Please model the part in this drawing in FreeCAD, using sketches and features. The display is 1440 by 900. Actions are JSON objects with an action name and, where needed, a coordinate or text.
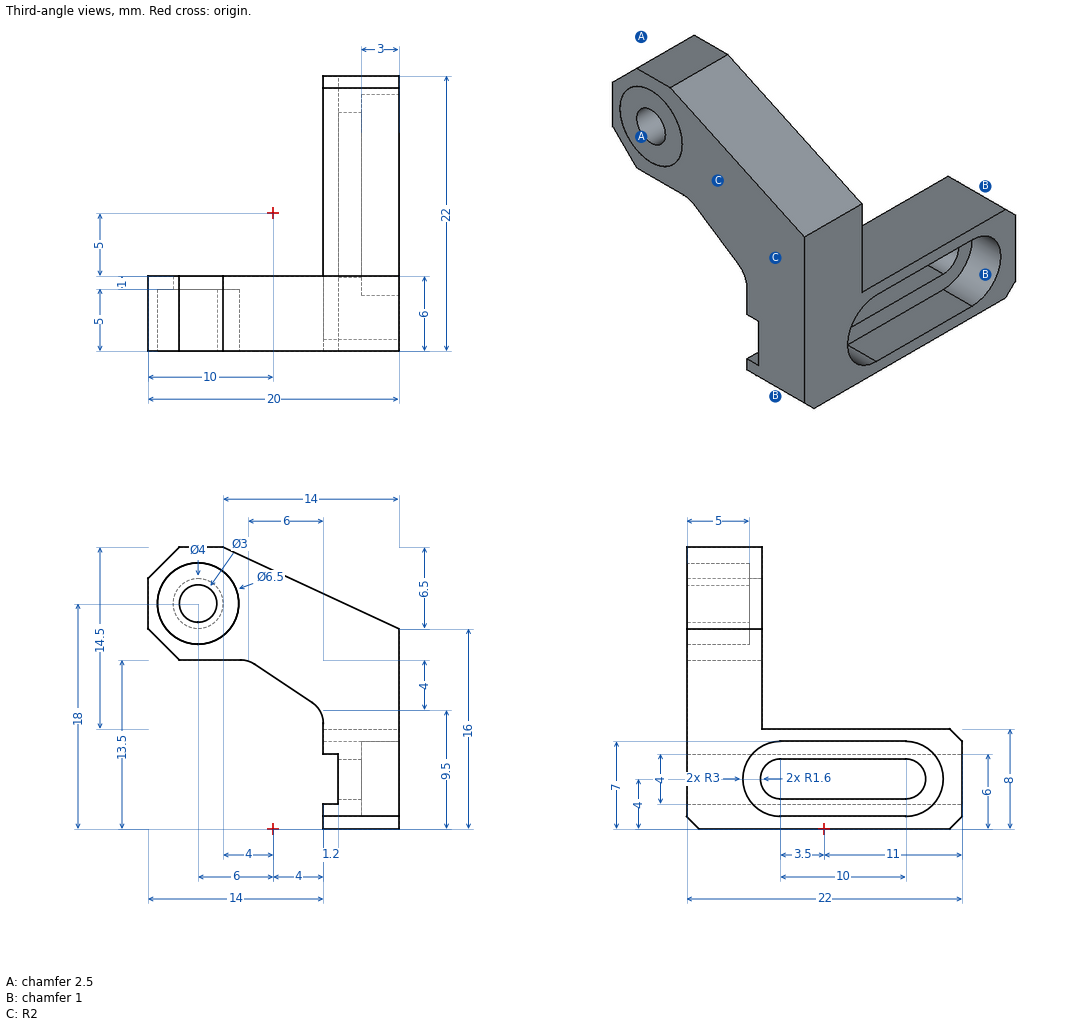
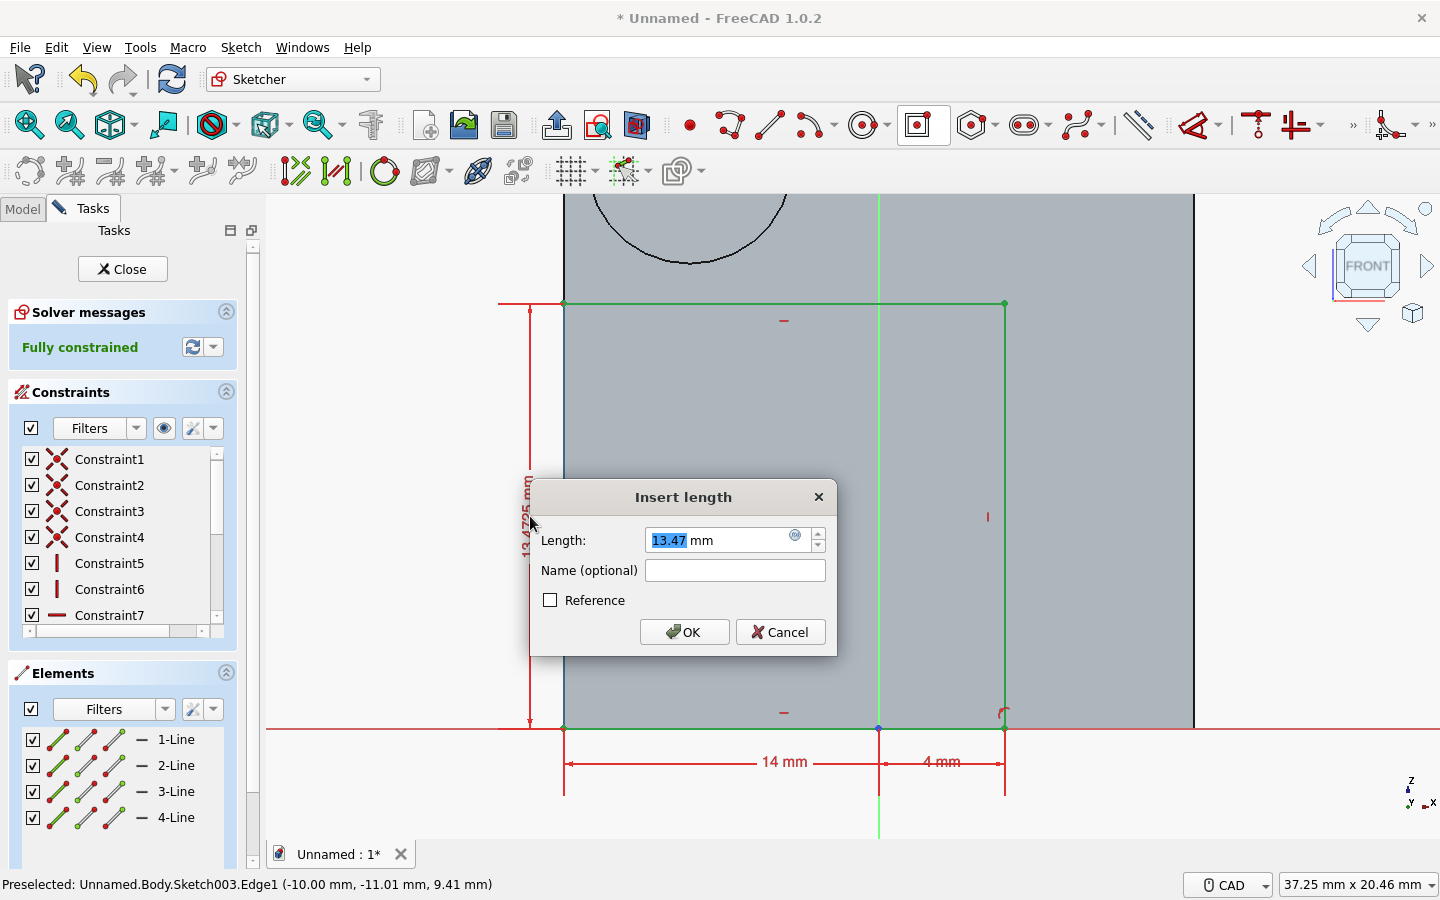
{"action": "type", "text": "13.5"}
{"action": "key", "text": "Return"}
{"action": "key", "text": "Escape"}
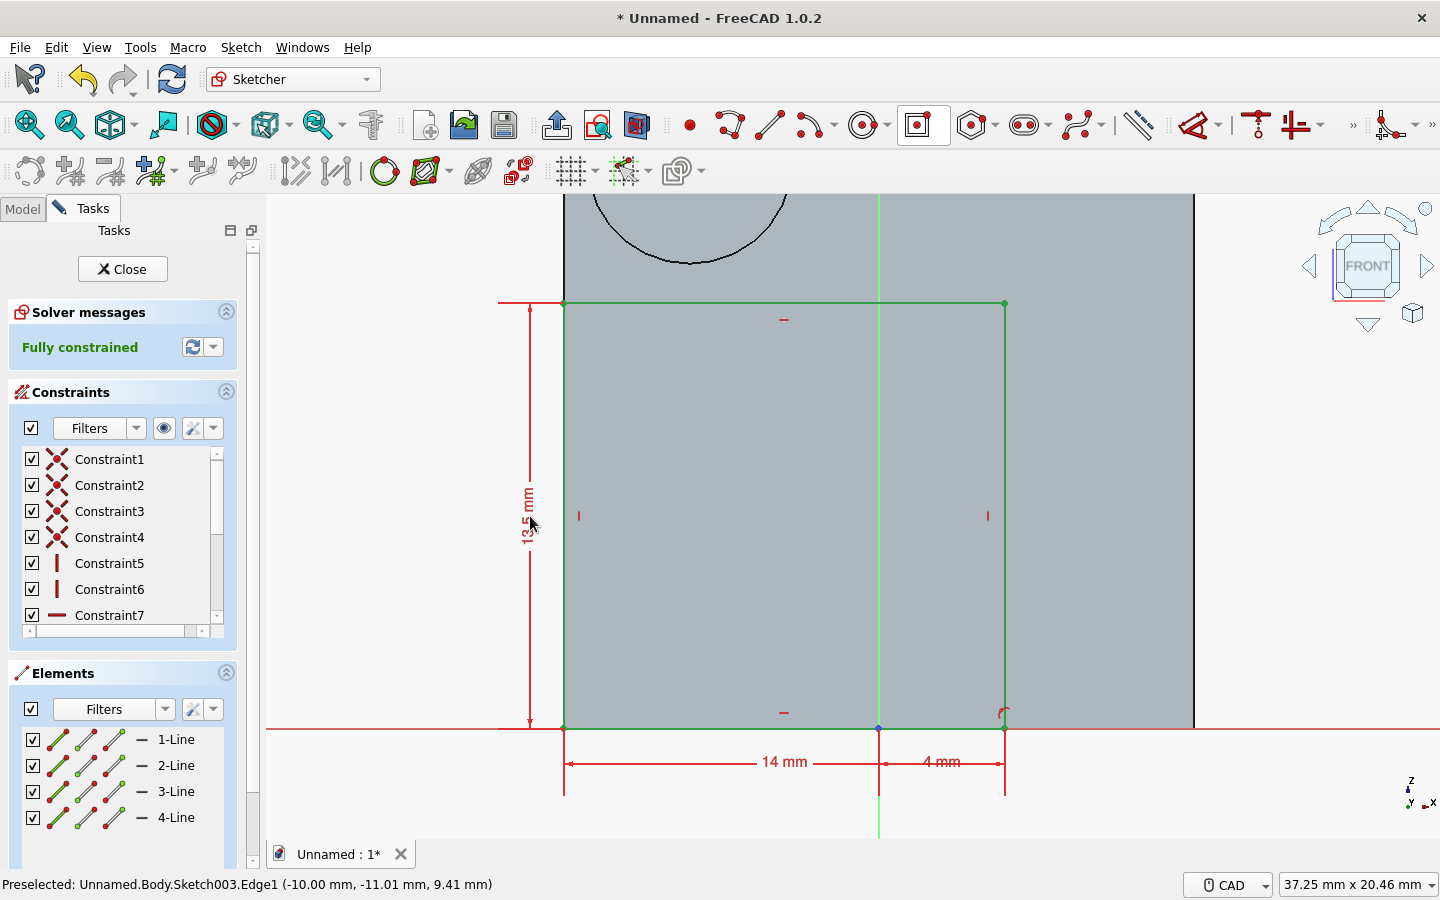
{"action": "left_click", "coordinate": [123, 269]}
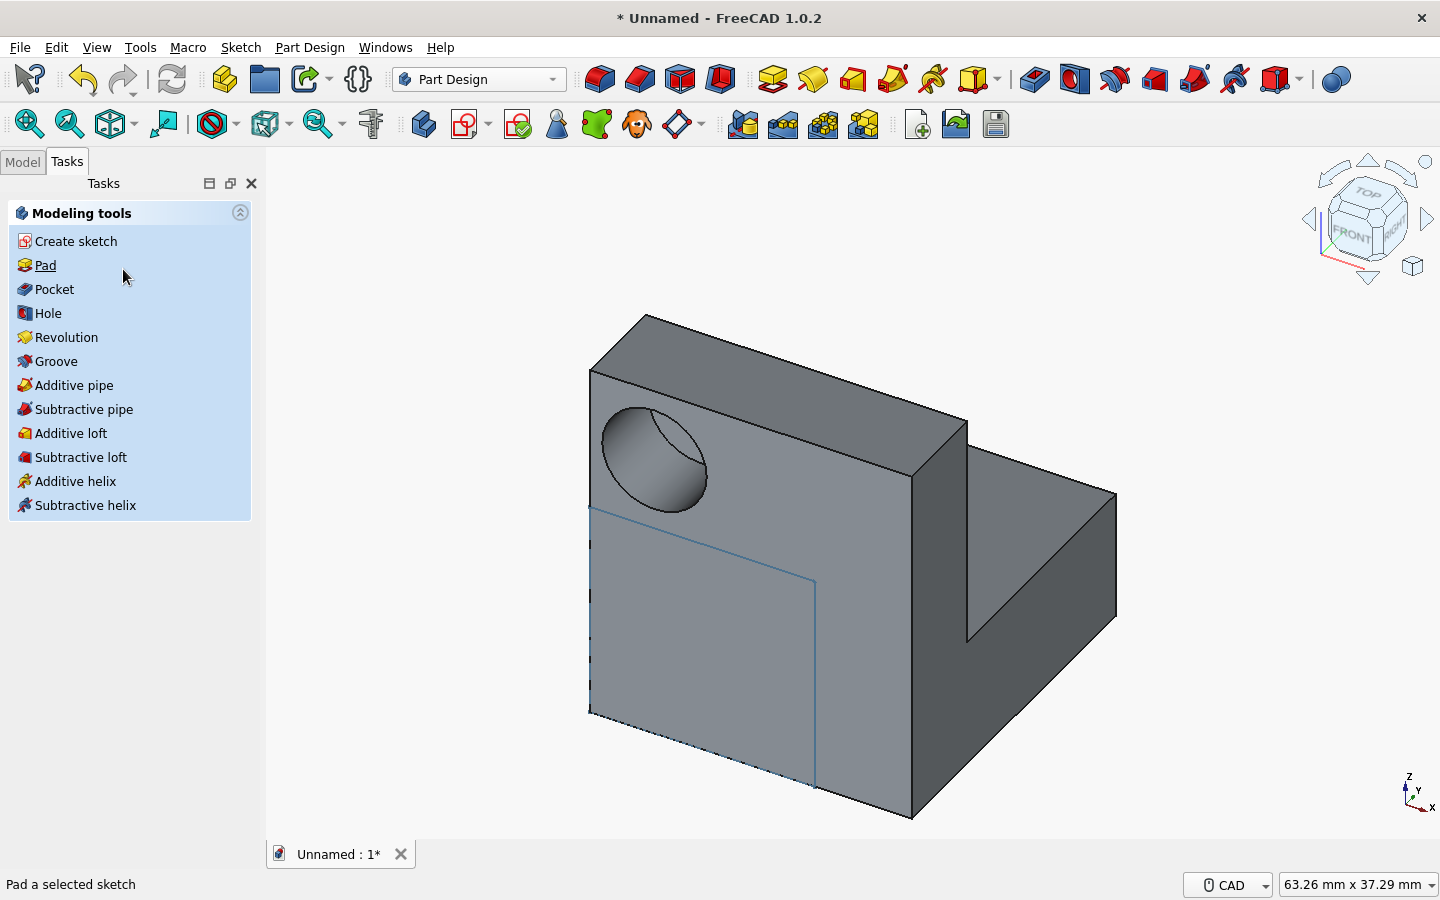
{"action": "left_click", "coordinate": [1036, 80]}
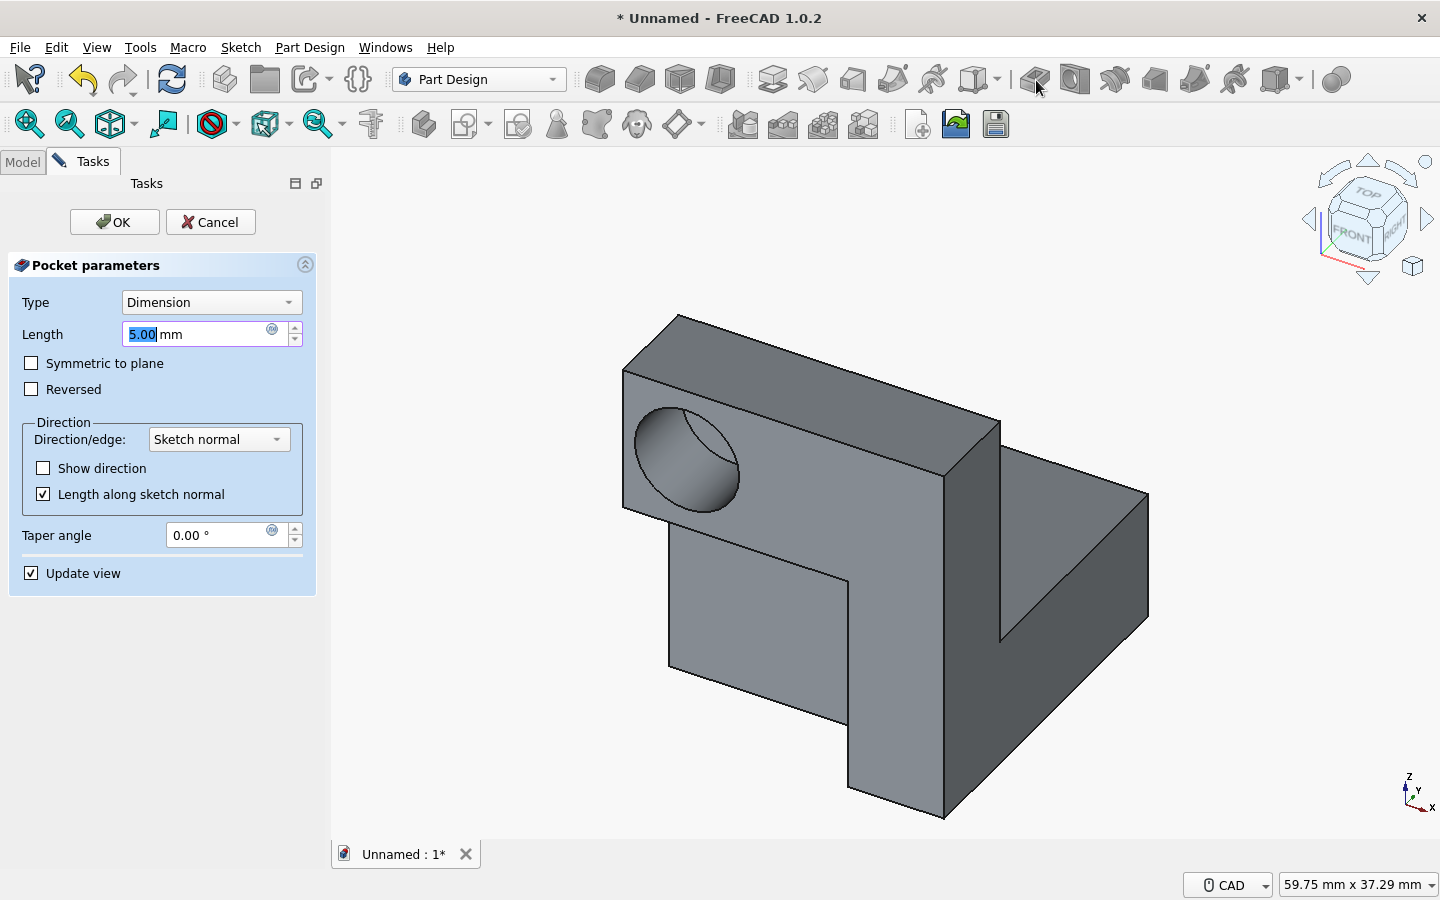
{"action": "left_click", "coordinate": [212, 302]}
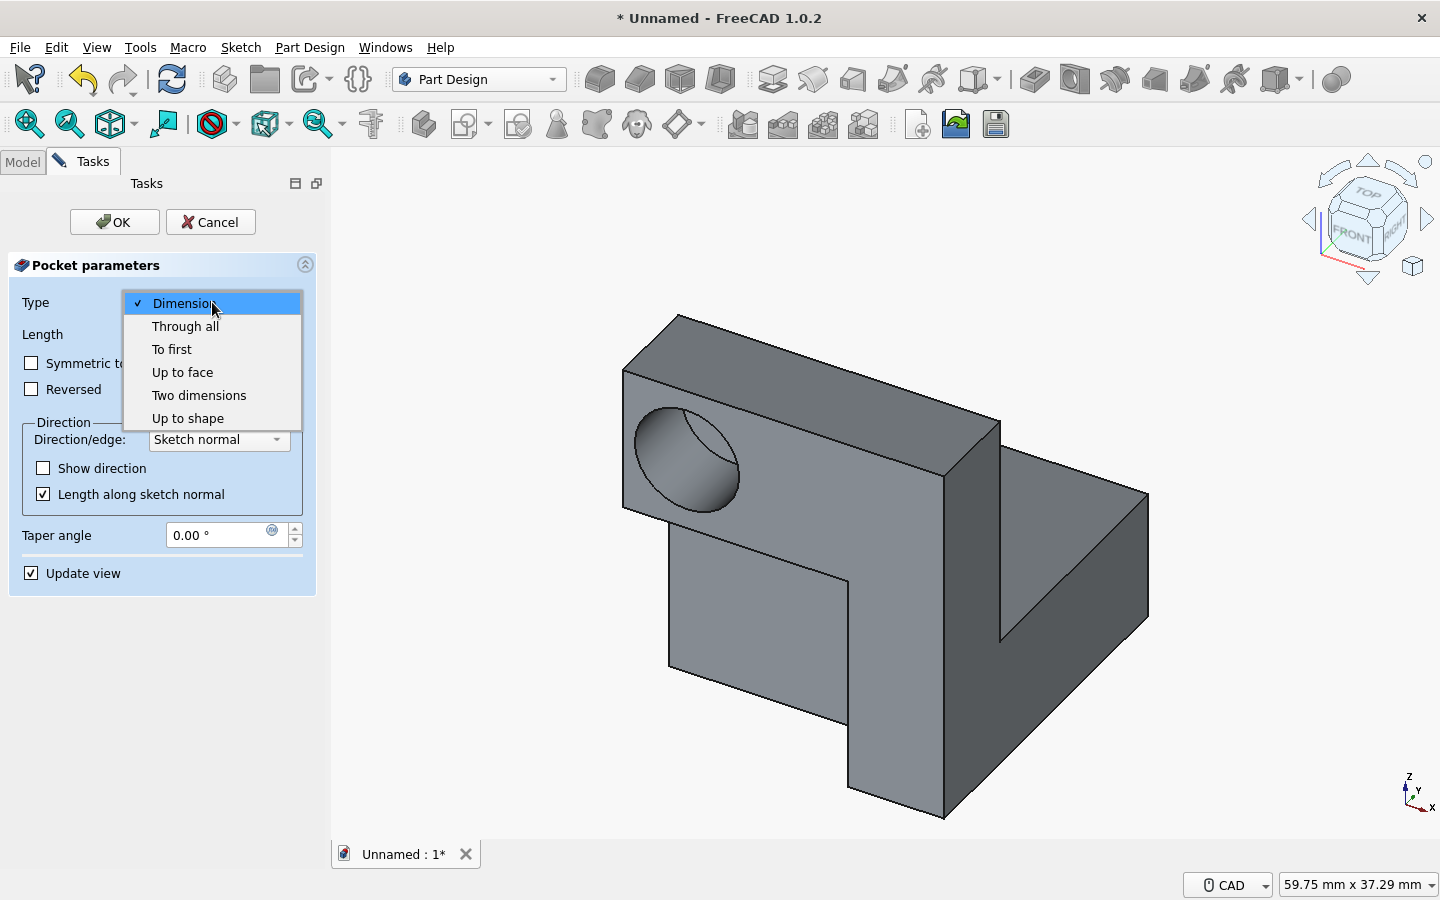
{"action": "left_click", "coordinate": [212, 326]}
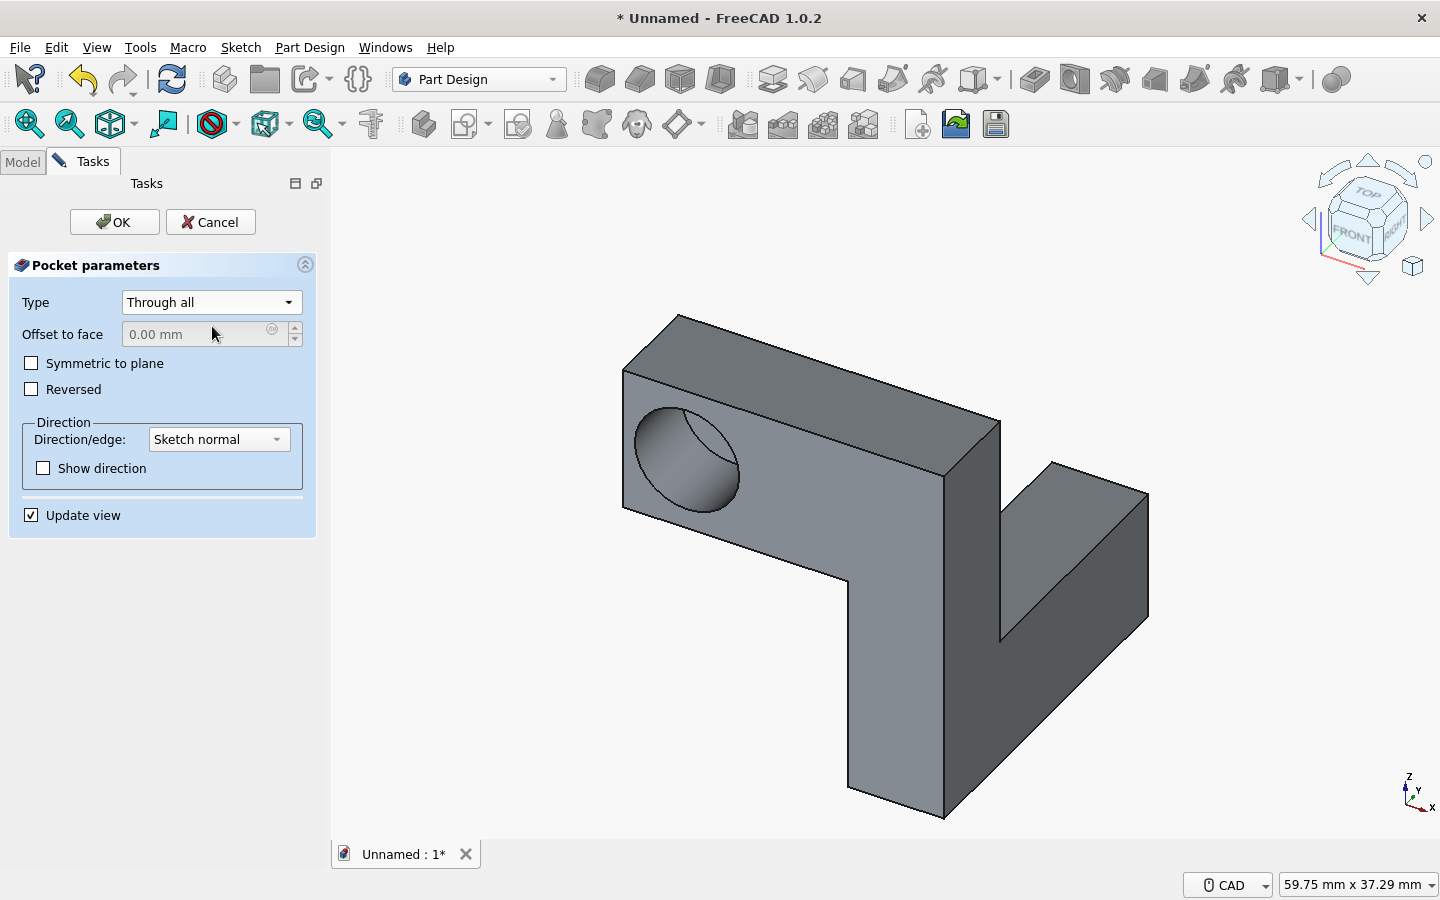
{"action": "left_click", "coordinate": [115, 222]}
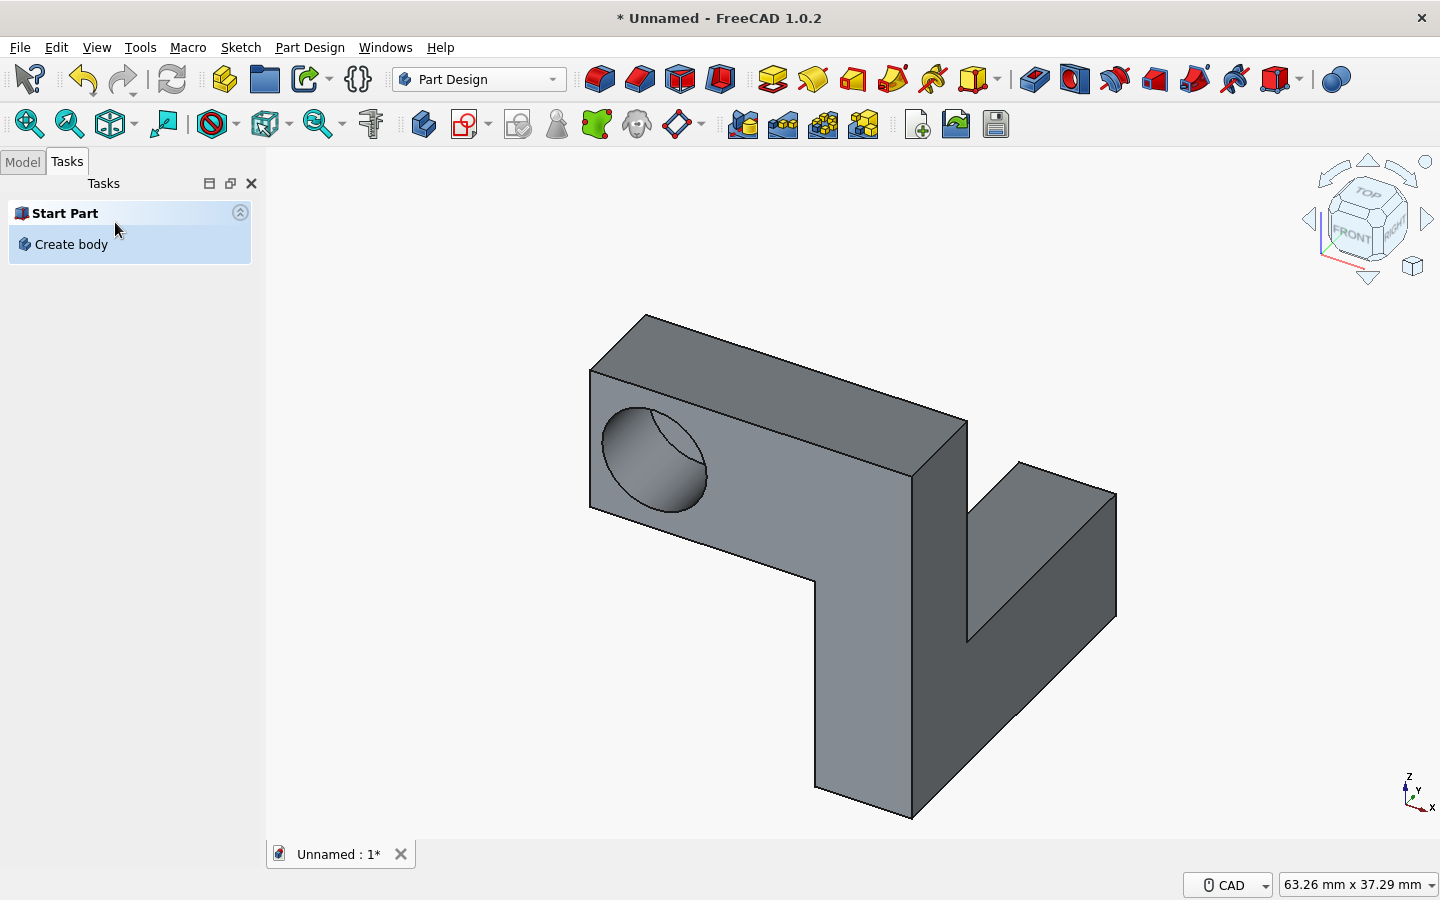
{"action": "key", "text": "6"}